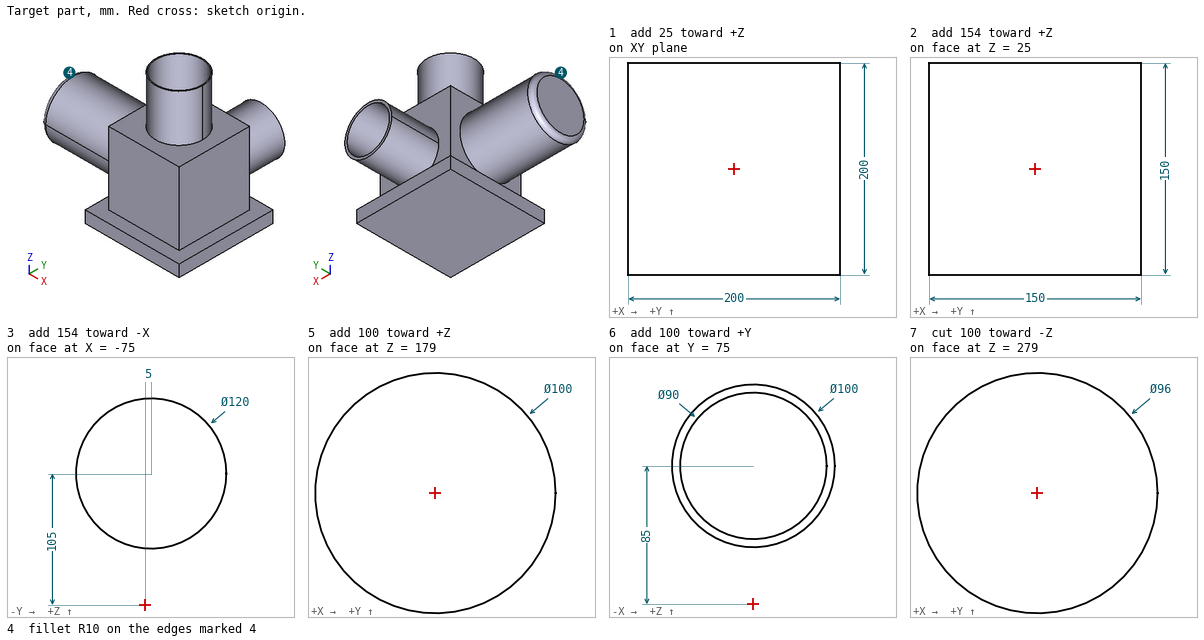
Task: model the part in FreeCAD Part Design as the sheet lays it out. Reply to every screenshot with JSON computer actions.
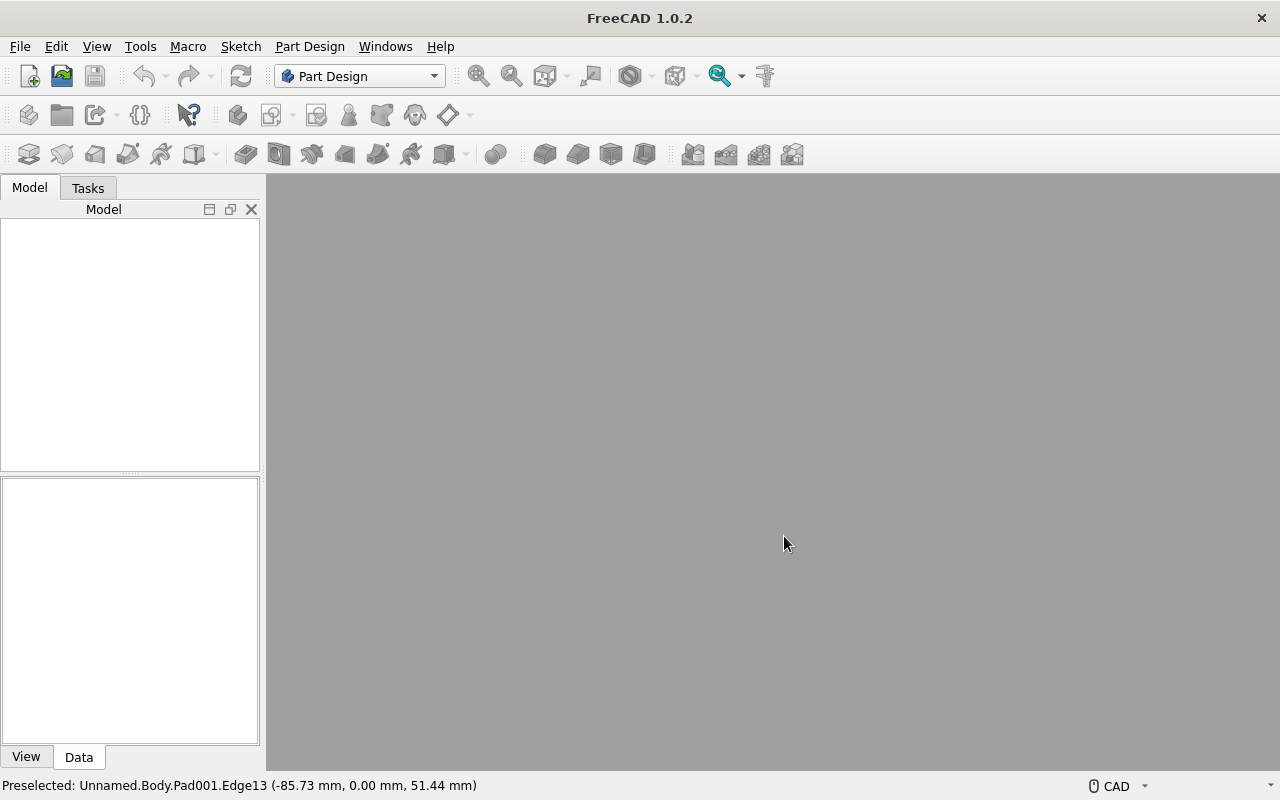
{"action": "left_click", "coordinate": [29, 76]}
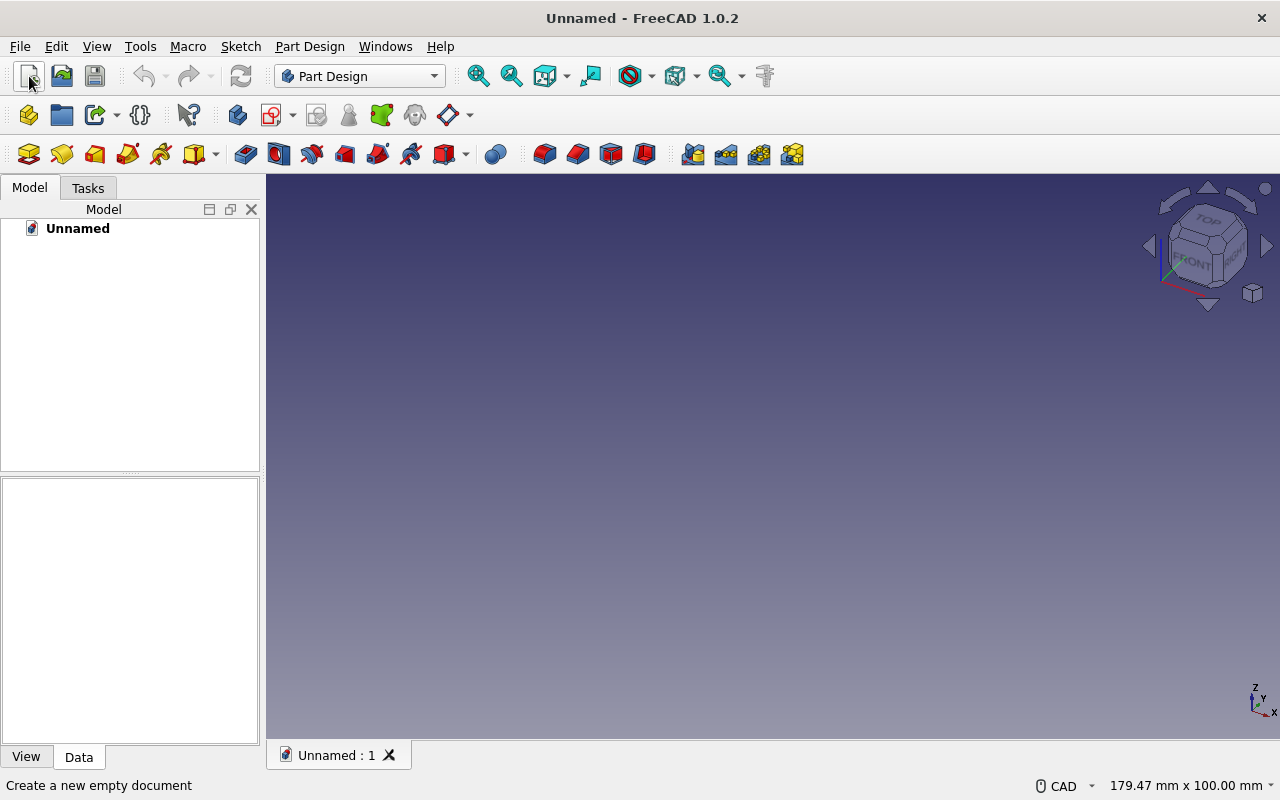
{"action": "left_click", "coordinate": [270, 116]}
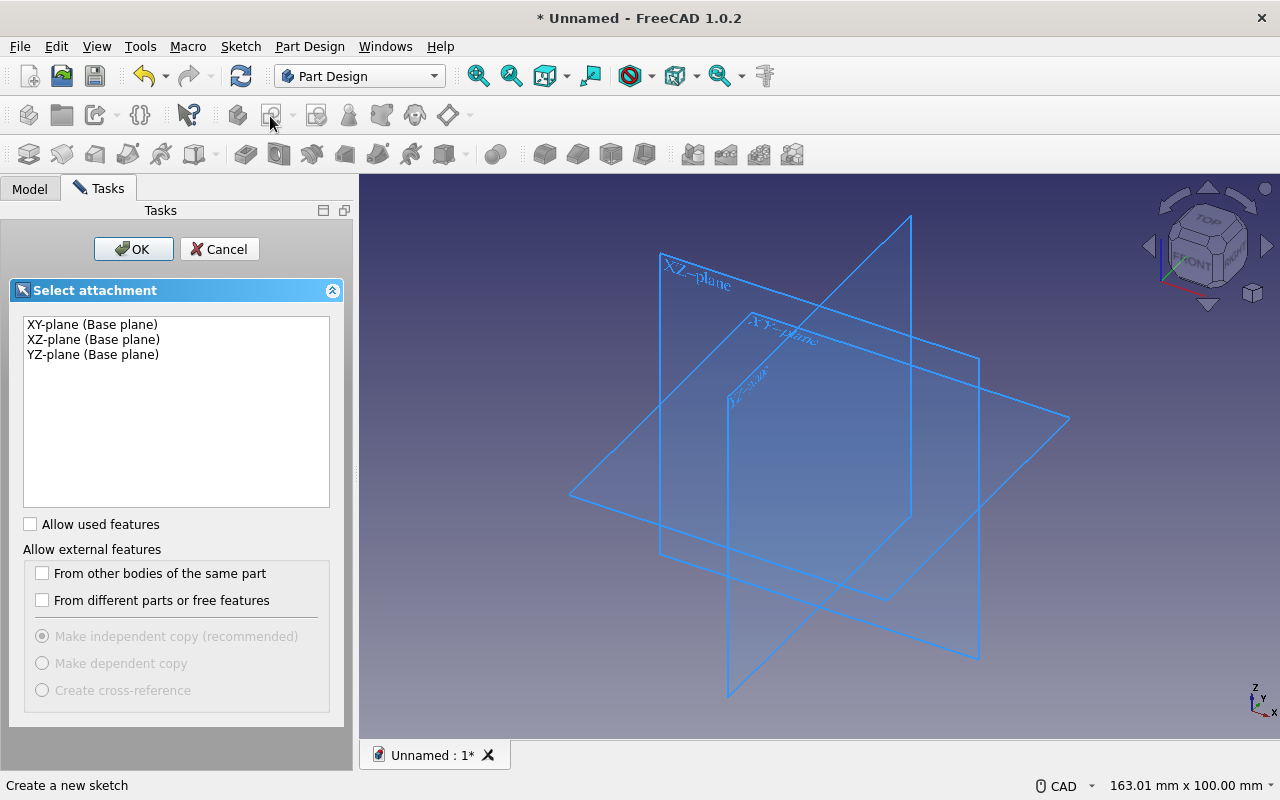
{"action": "left_click", "coordinate": [84, 324]}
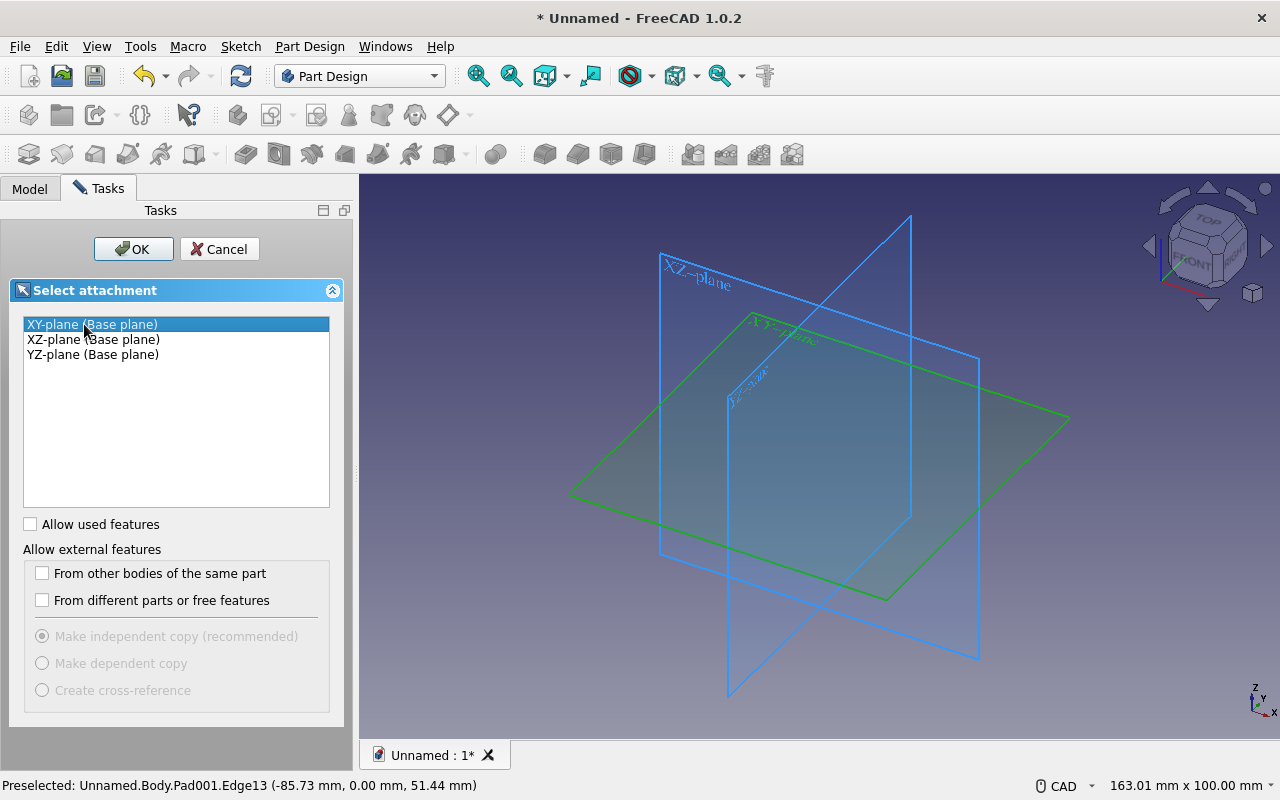
{"action": "left_click", "coordinate": [134, 249]}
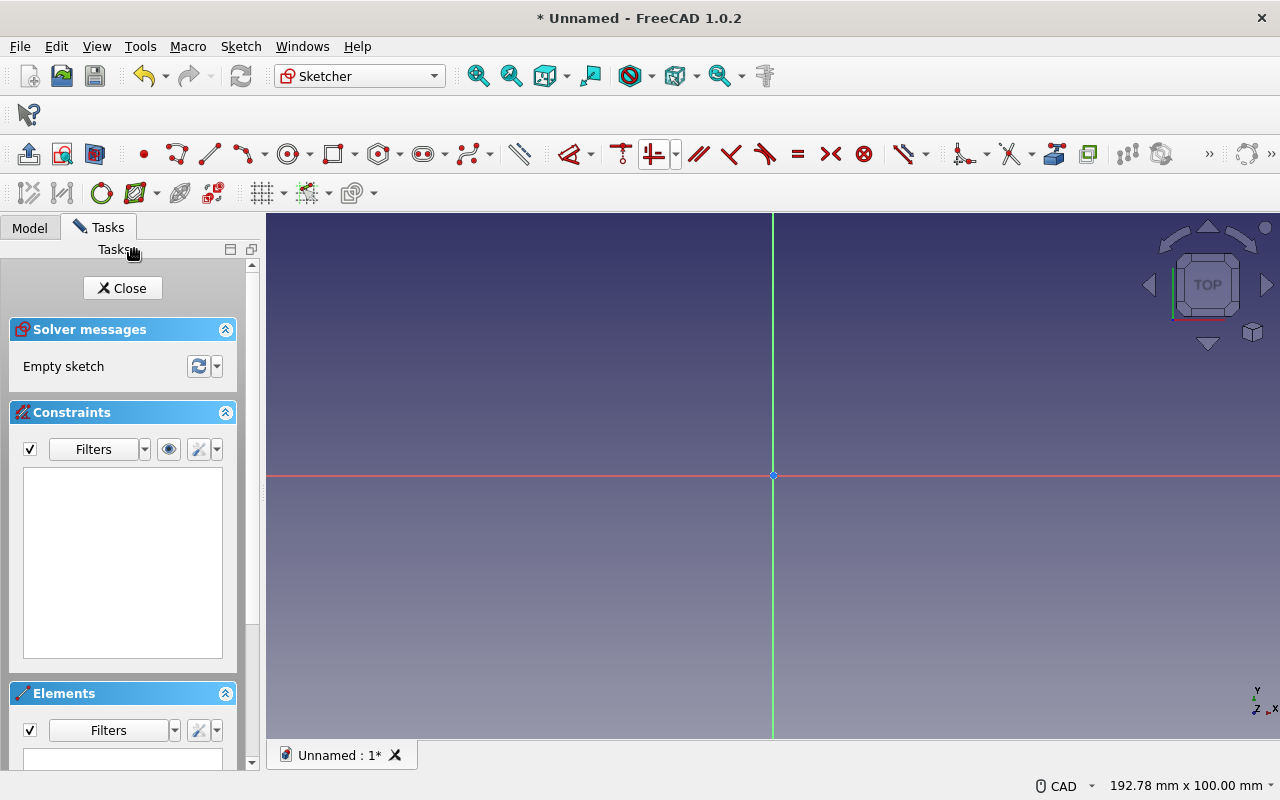
{"action": "scroll", "coordinate": [675, 476], "scroll_direction": "down", "scroll_amount": 6}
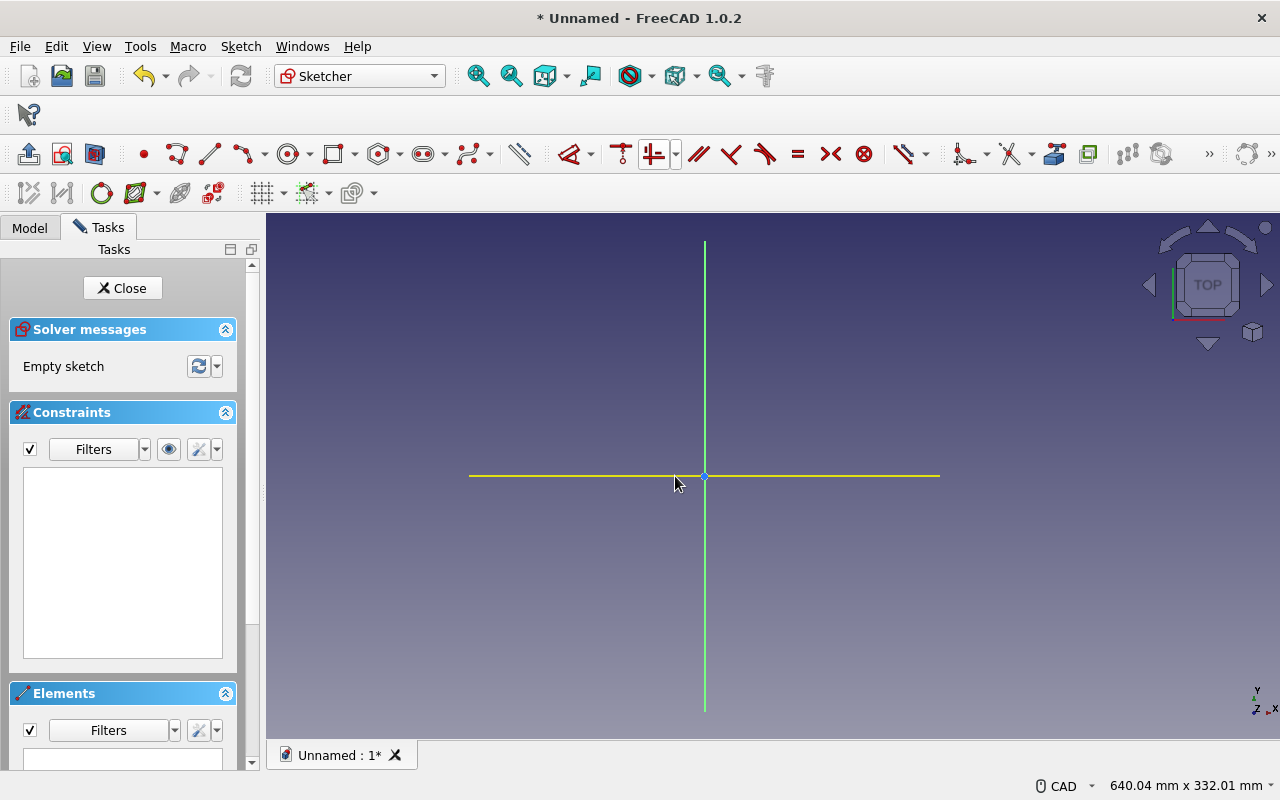
{"action": "left_click", "coordinate": [354, 154]}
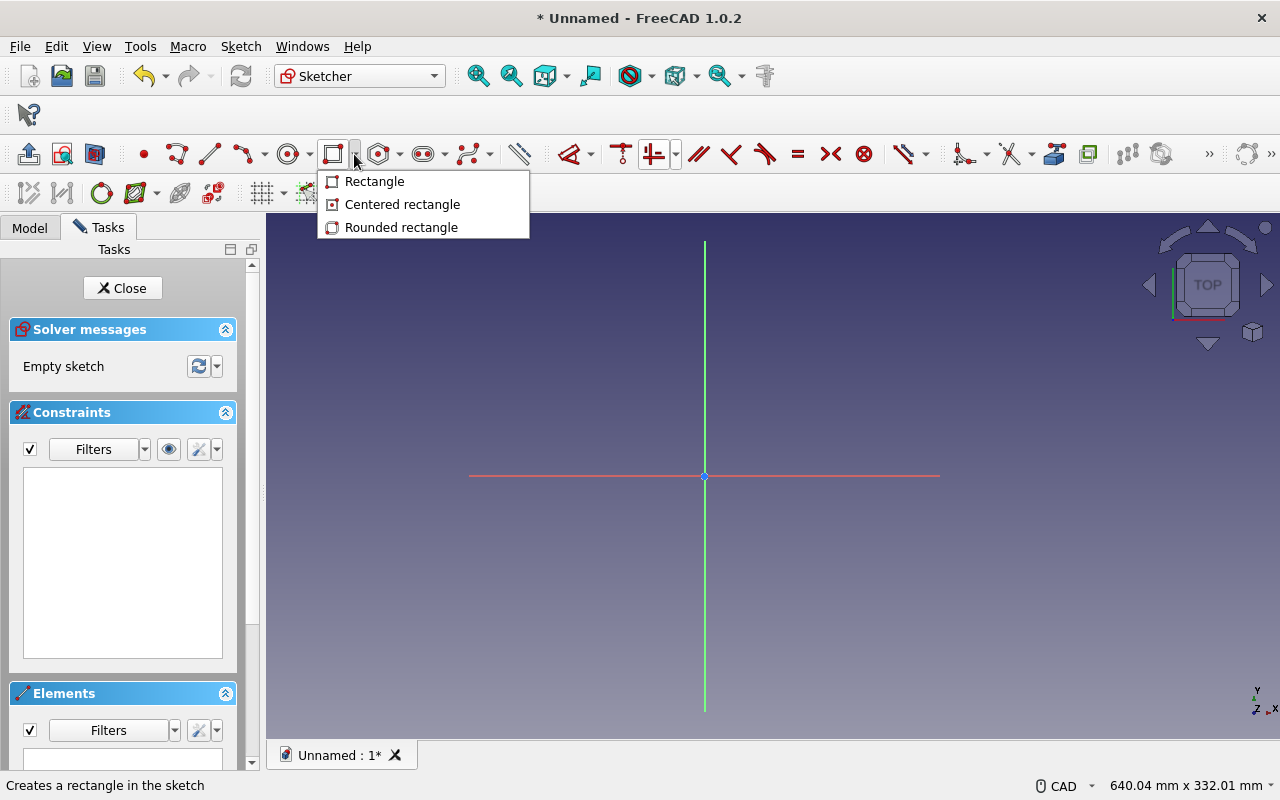
{"action": "left_click", "coordinate": [424, 204]}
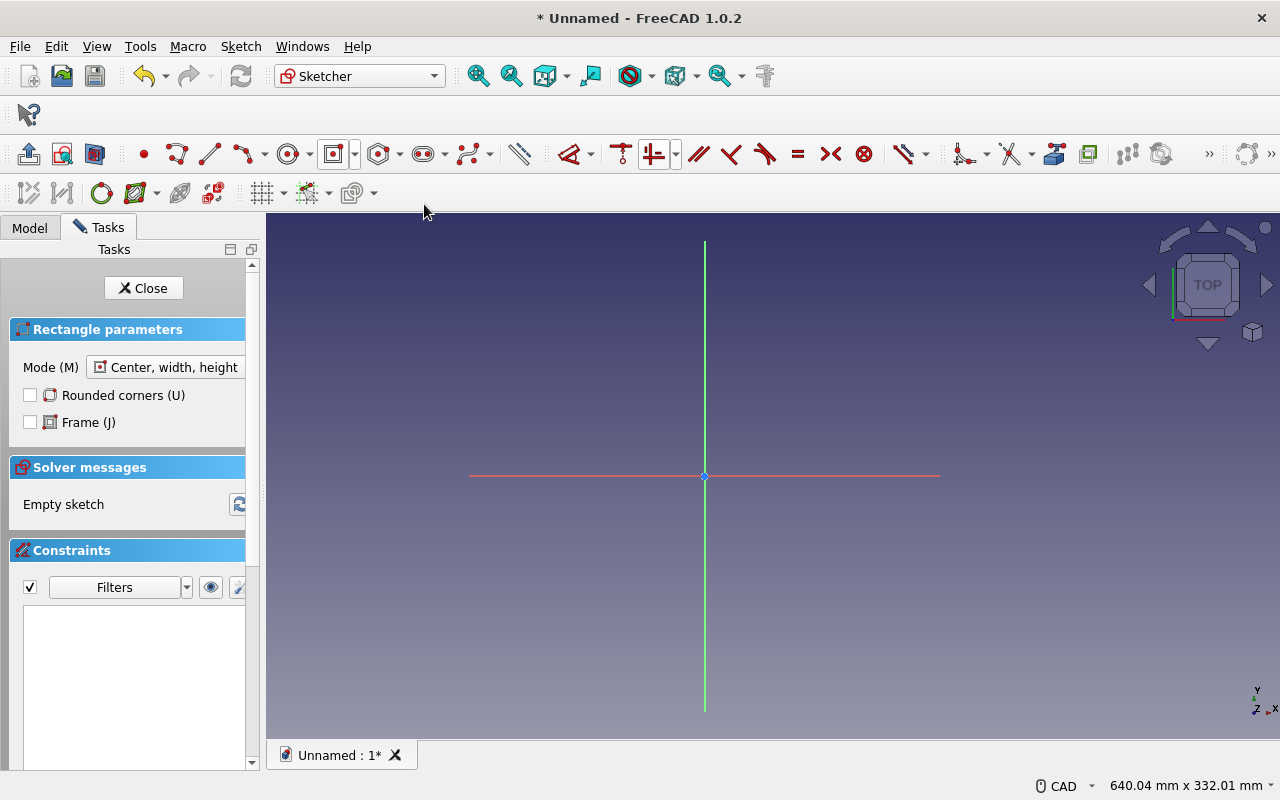
{"action": "left_click", "coordinate": [705, 476]}
{"action": "mouse_move", "coordinate": [863, 318]}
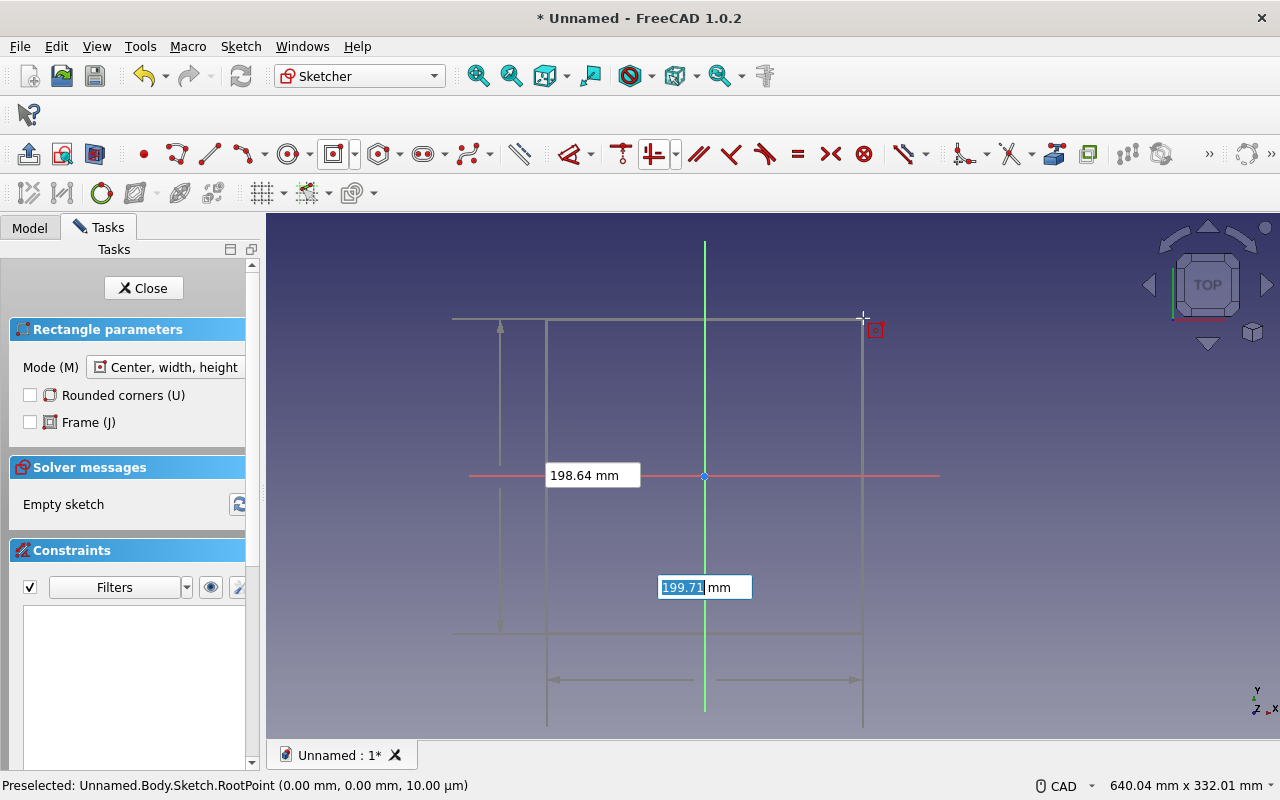
{"action": "type", "text": "200"}
{"action": "key", "text": "Tab"}
{"action": "type", "text": "200"}
{"action": "key", "text": "Return"}
{"action": "key", "text": "Escape"}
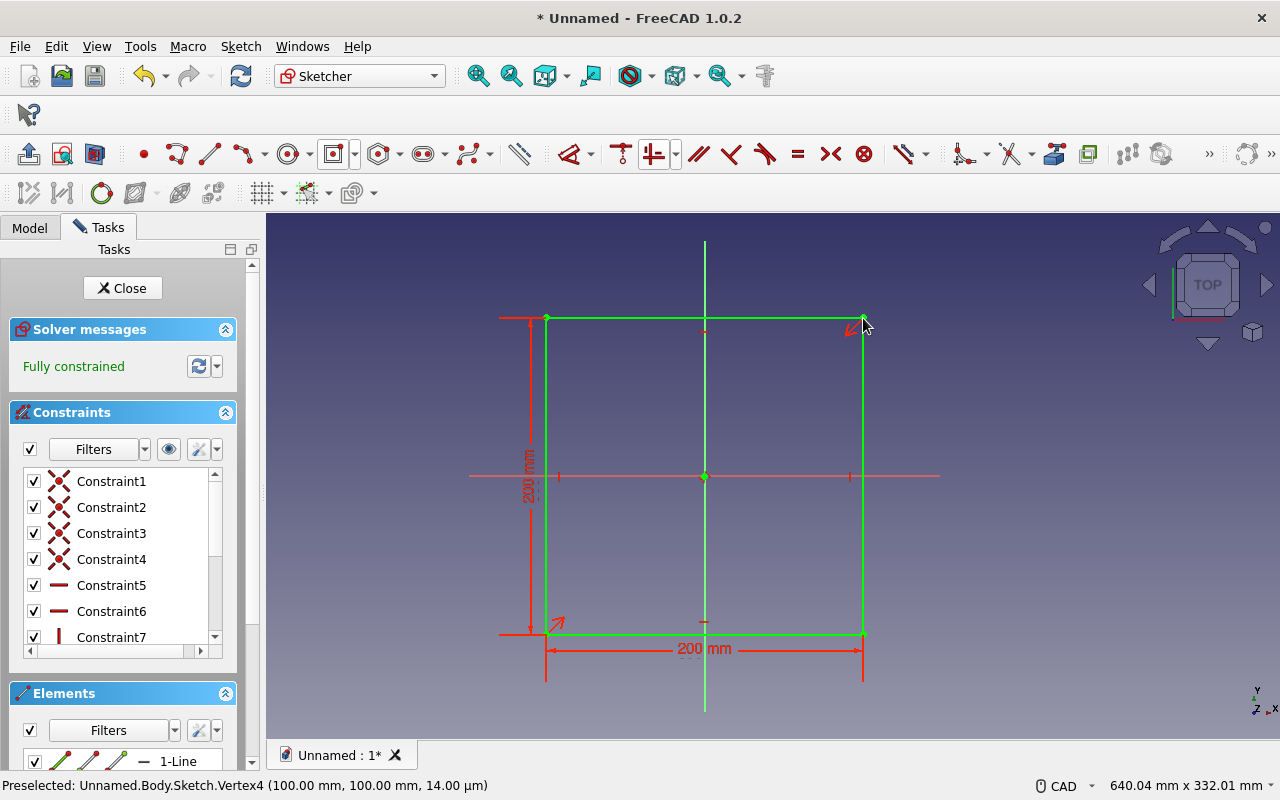
{"action": "left_click", "coordinate": [123, 288]}